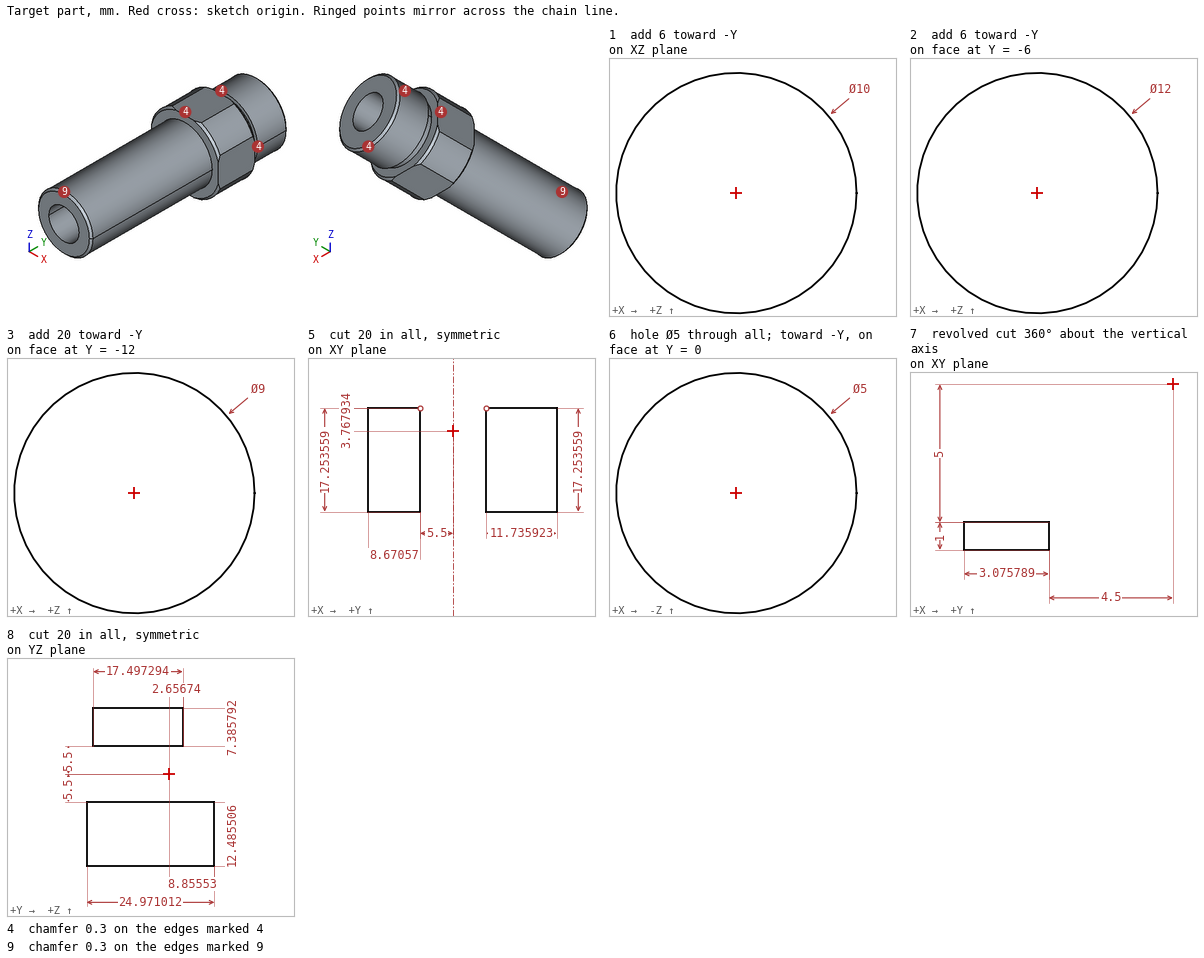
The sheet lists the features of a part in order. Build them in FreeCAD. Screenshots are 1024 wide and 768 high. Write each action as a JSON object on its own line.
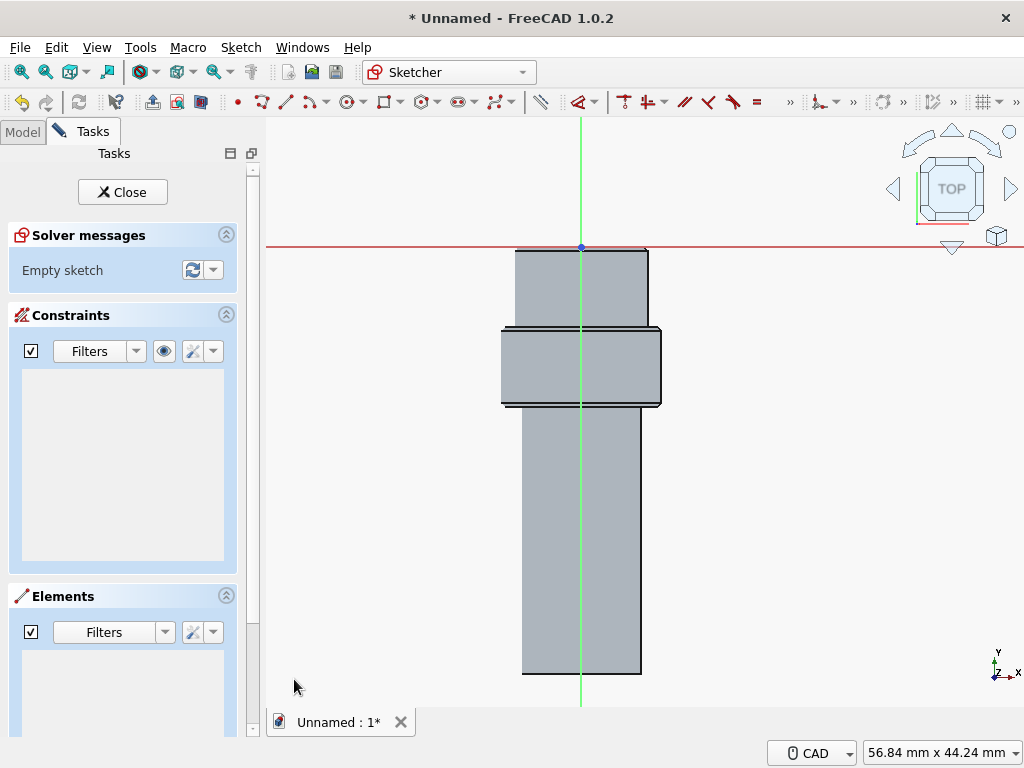
{"action": "key", "text": "g r"}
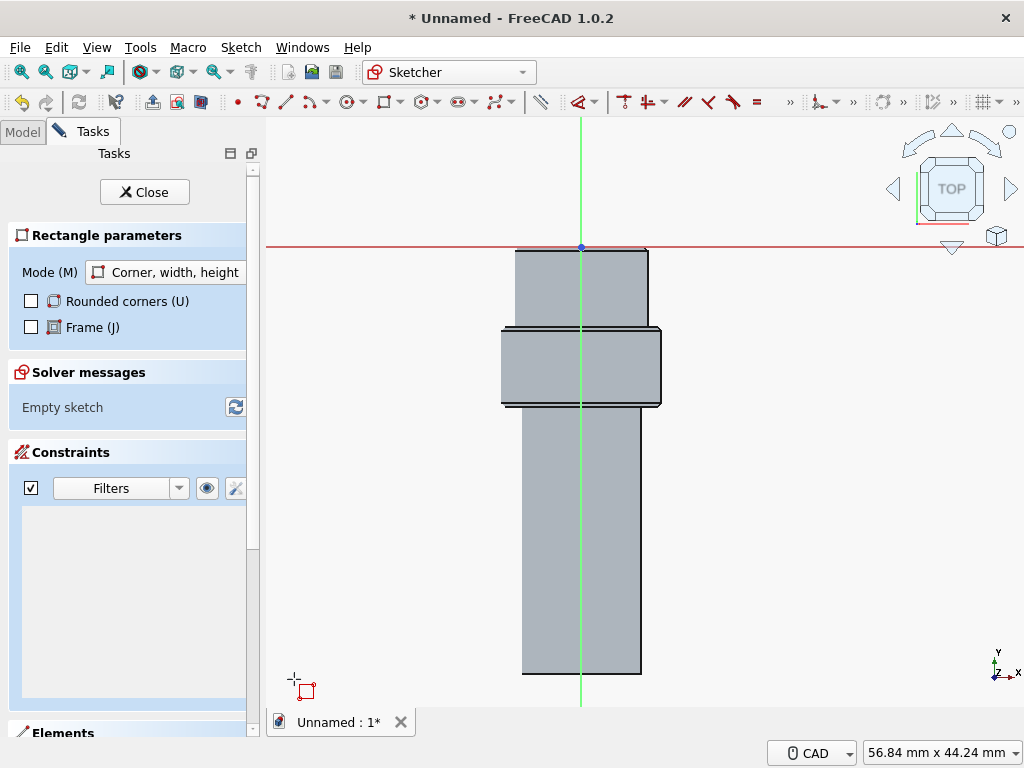
{"action": "left_click", "coordinate": [392, 197]}
{"action": "mouse_move", "coordinate": [508, 427]}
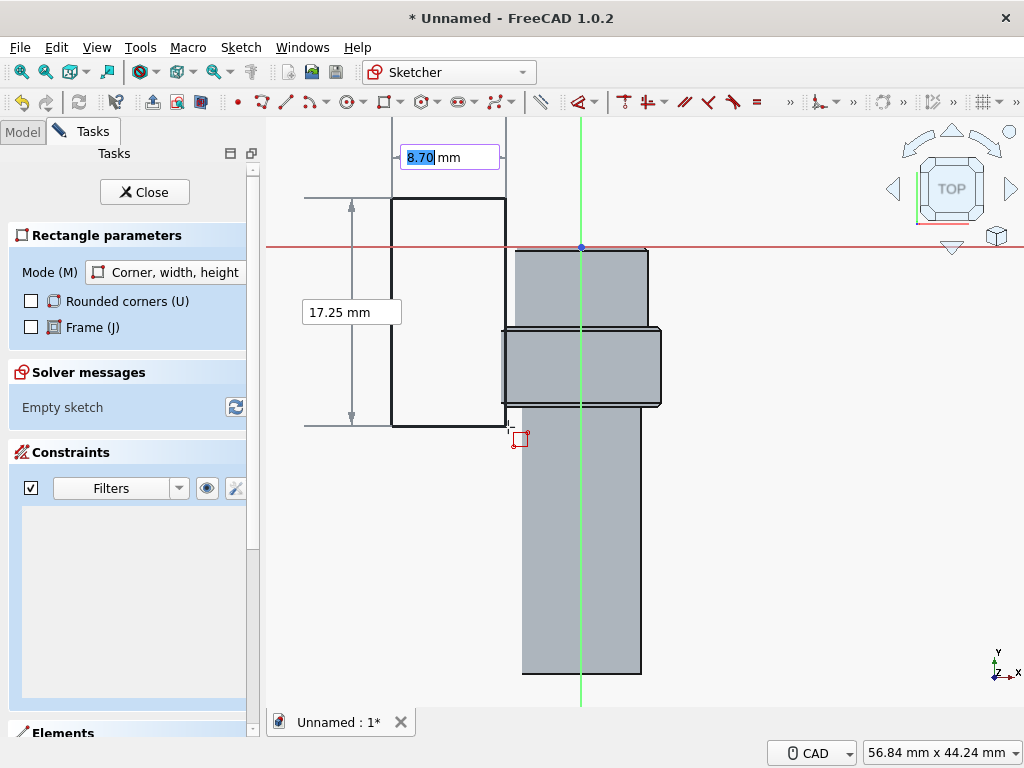
{"action": "type", "text": "8.67057"}
{"action": "key", "text": "Tab"}
{"action": "type", "text": "17.253559"}
{"action": "key", "text": "Return"}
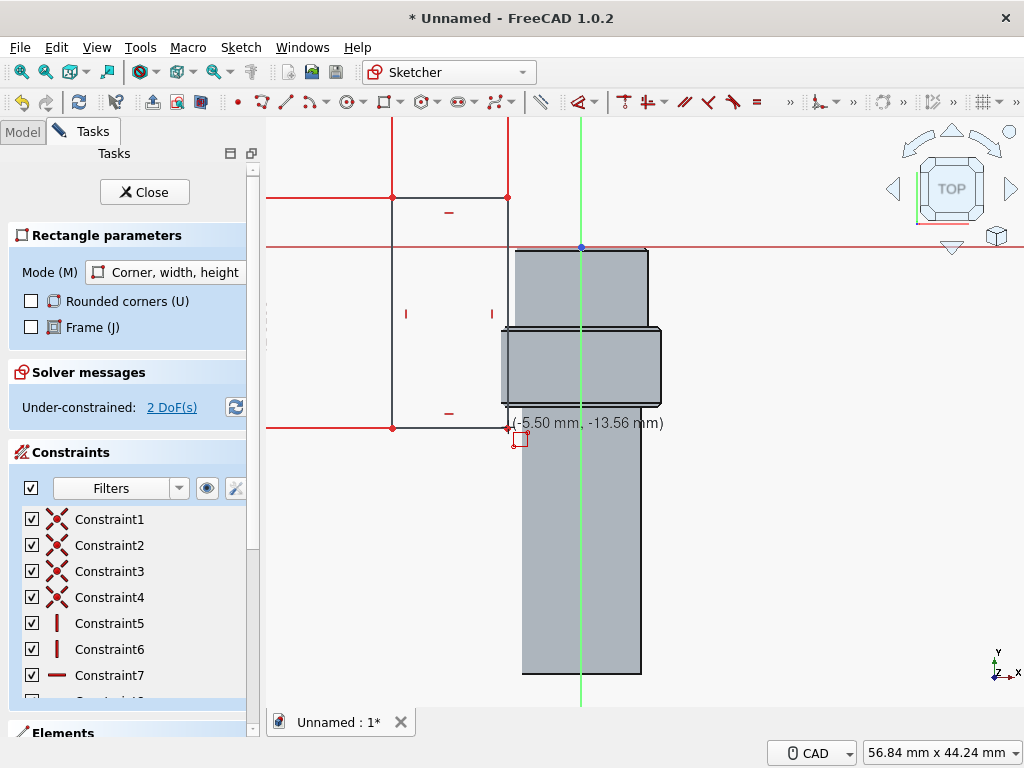
{"action": "left_click", "coordinate": [655, 197]}
{"action": "mouse_move", "coordinate": [811, 427]}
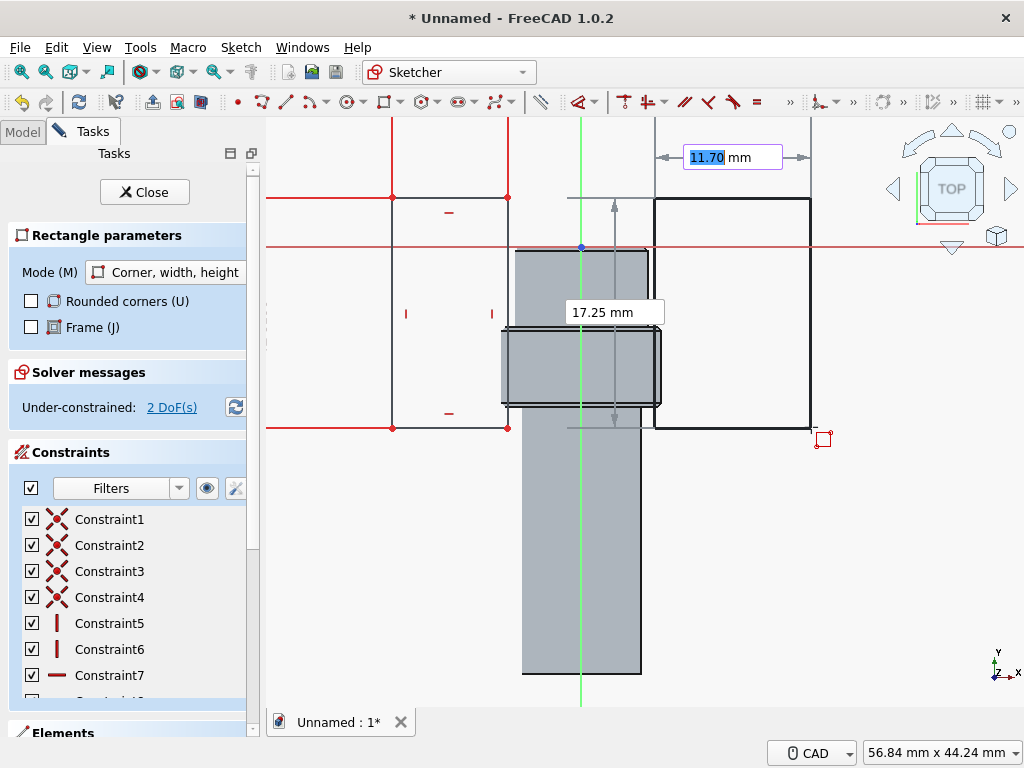
{"action": "type", "text": "11.735923"}
{"action": "key", "text": "Tab"}
{"action": "type", "text": "17.253559"}
{"action": "key", "text": "Return"}
{"action": "key", "text": "Escape"}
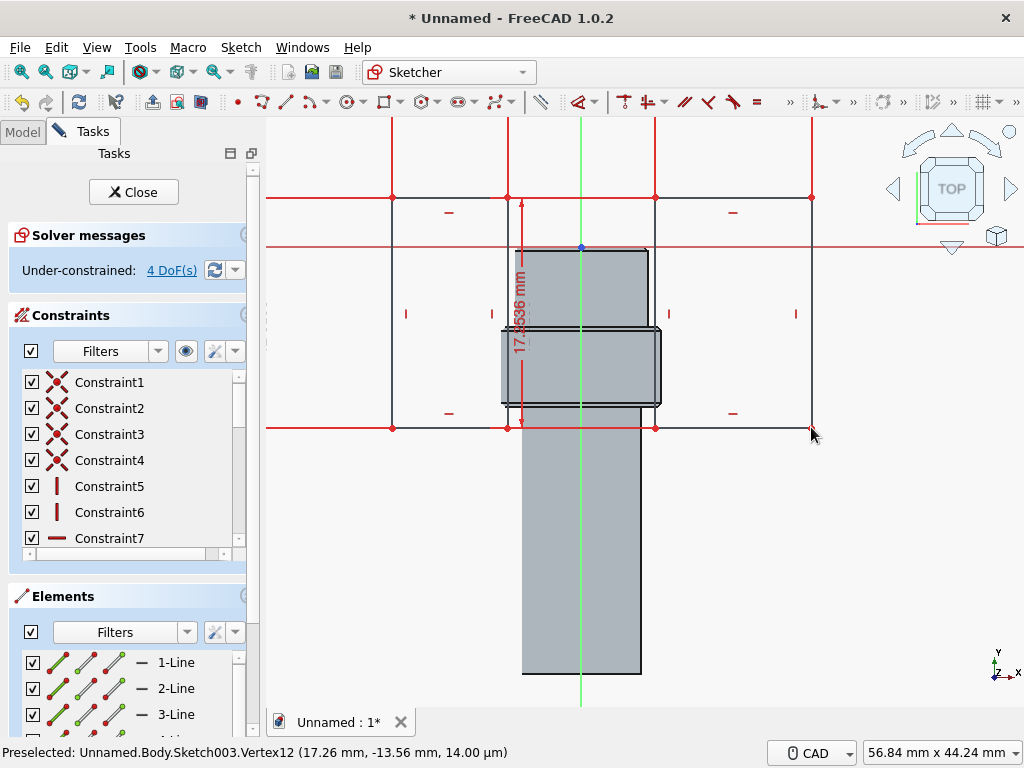
{"action": "left_click", "coordinate": [508, 198]}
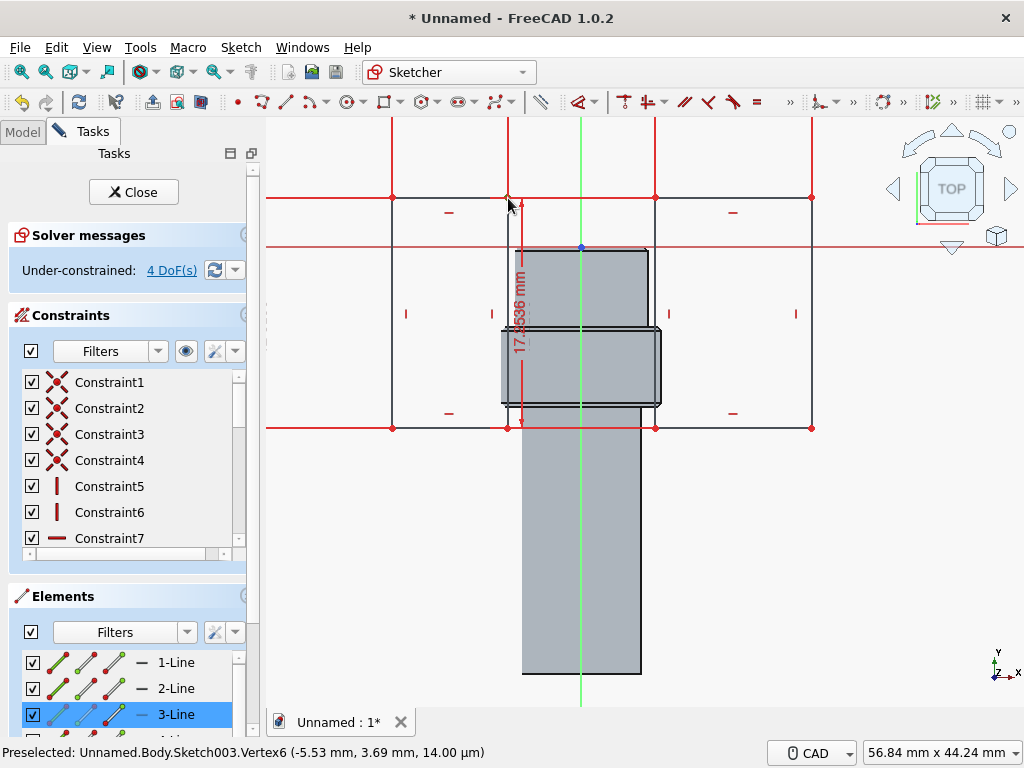
{"action": "left_click", "coordinate": [655, 198]}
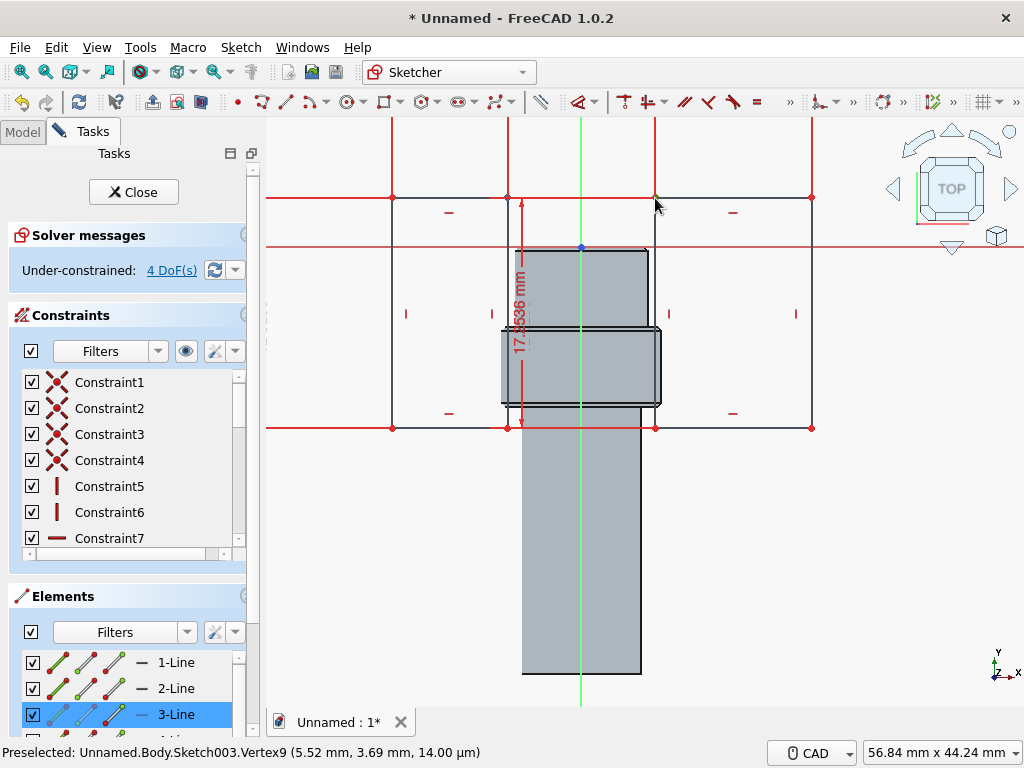
{"action": "left_click", "coordinate": [581, 641]}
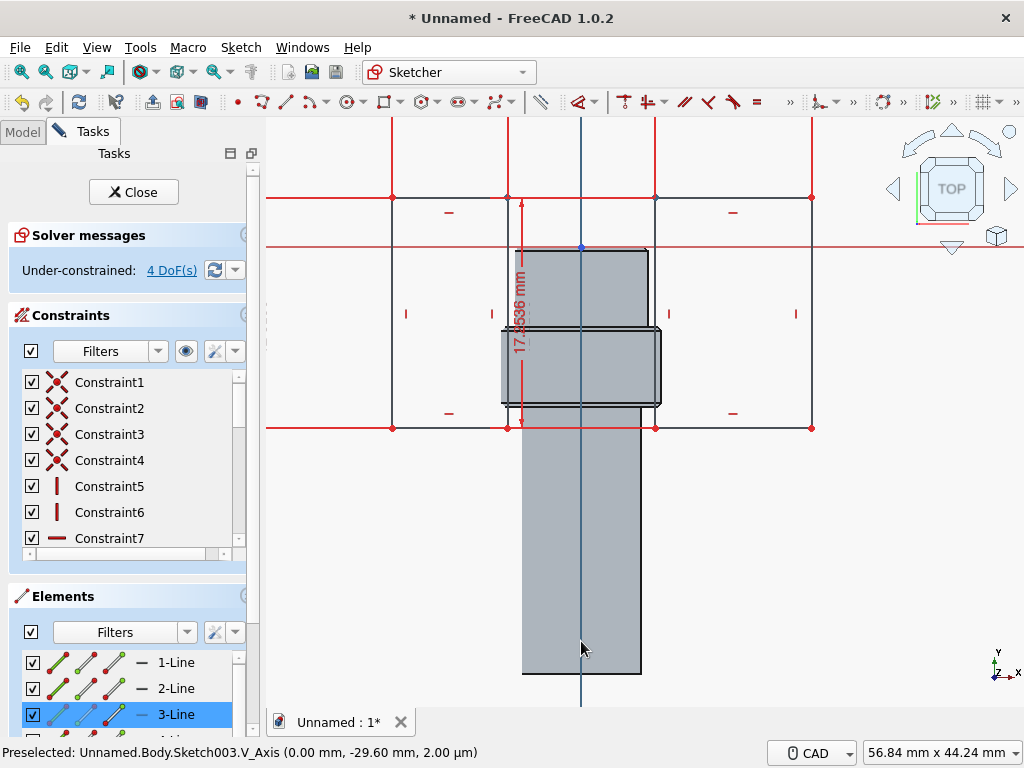
{"action": "key", "text": "s"}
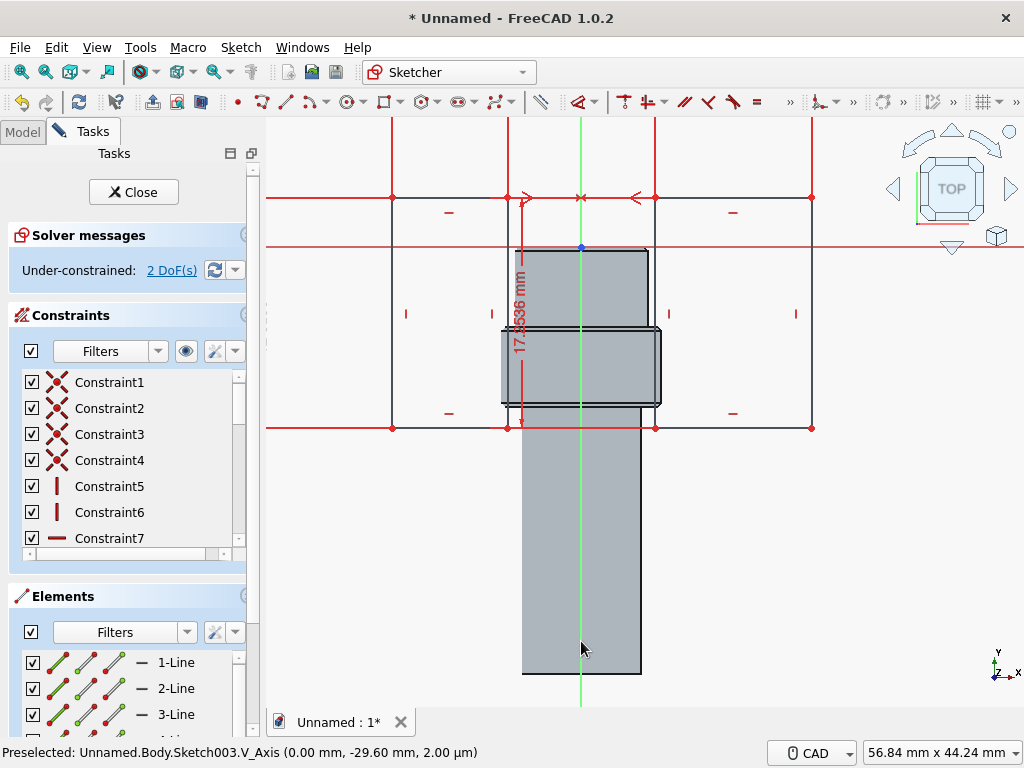
{"action": "left_click", "coordinate": [578, 102]}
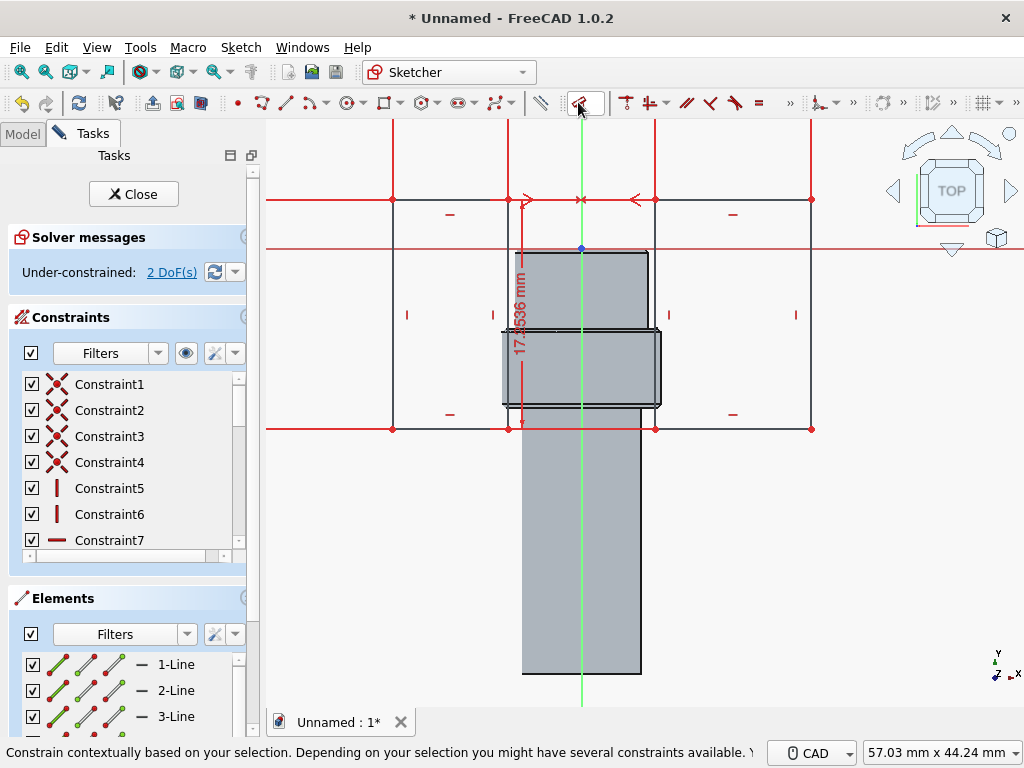
{"action": "left_click", "coordinate": [508, 429]}
{"action": "left_click", "coordinate": [545, 463]}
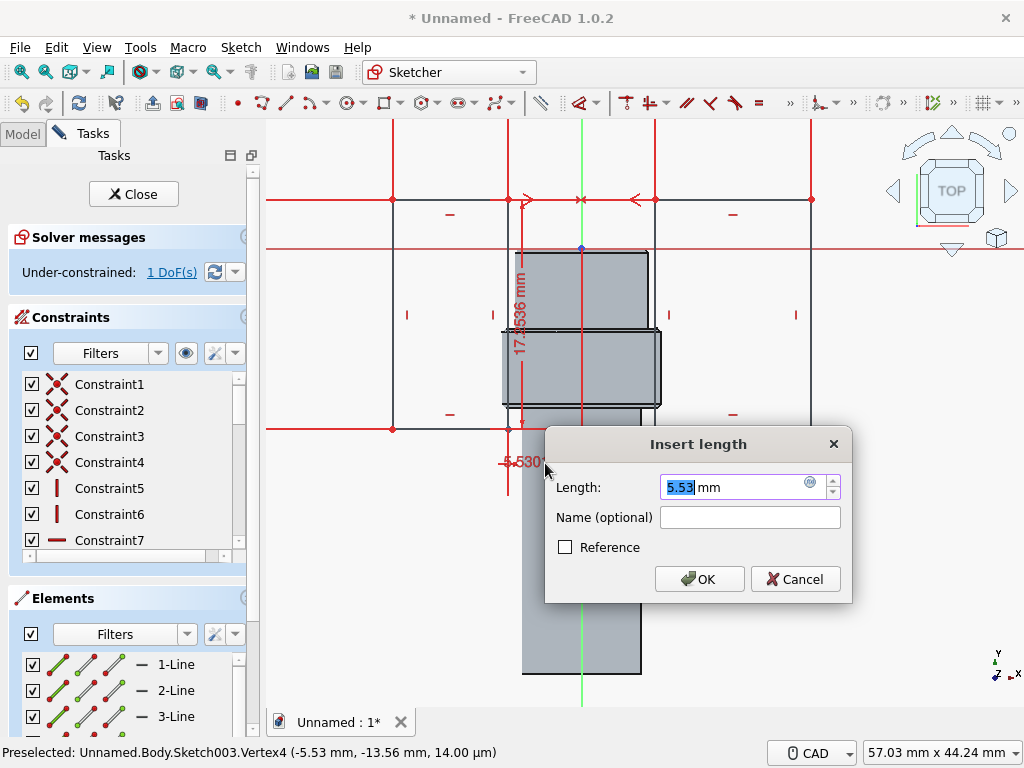
{"action": "type", "text": "5.5"}
{"action": "key", "text": "Return"}